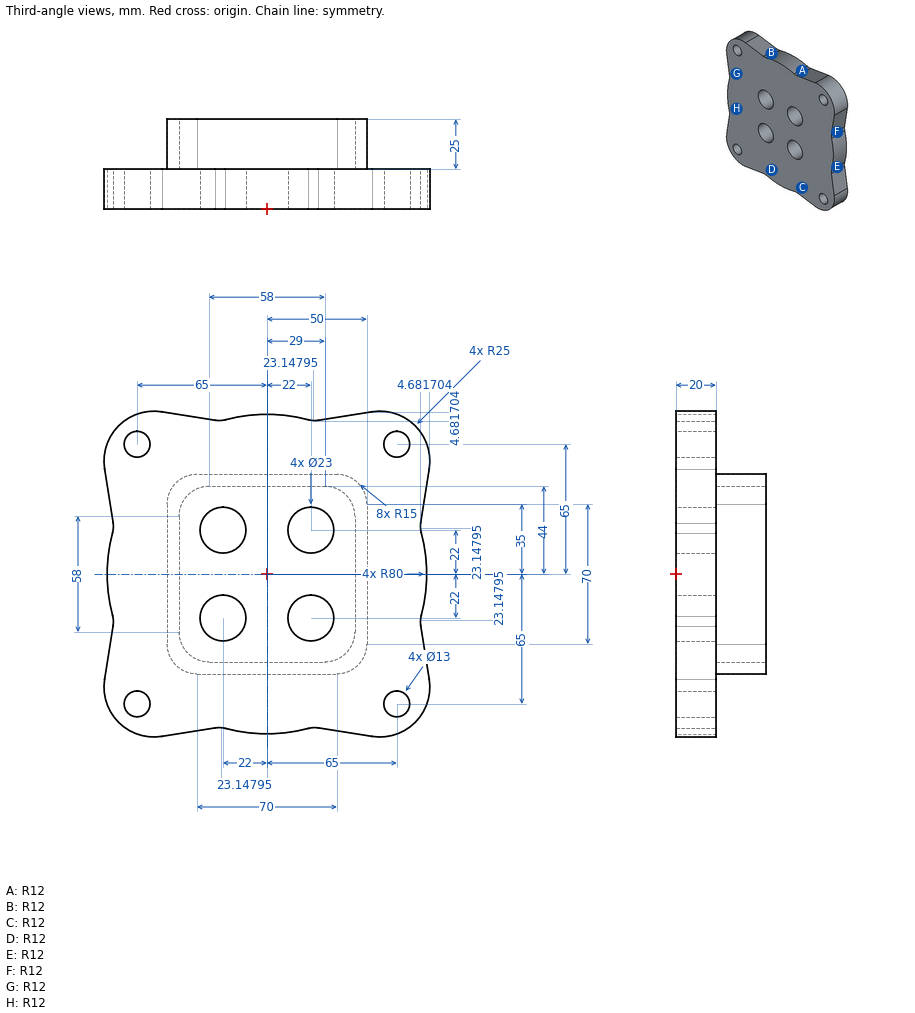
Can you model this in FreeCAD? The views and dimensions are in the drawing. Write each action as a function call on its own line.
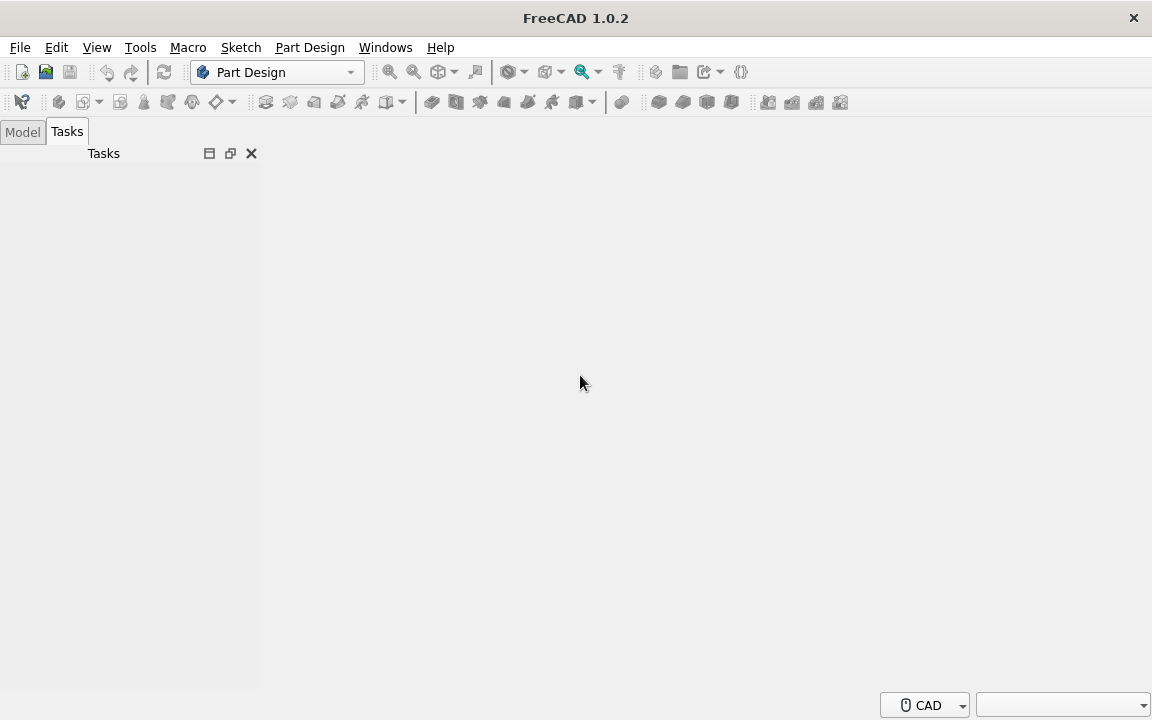
click(22, 72)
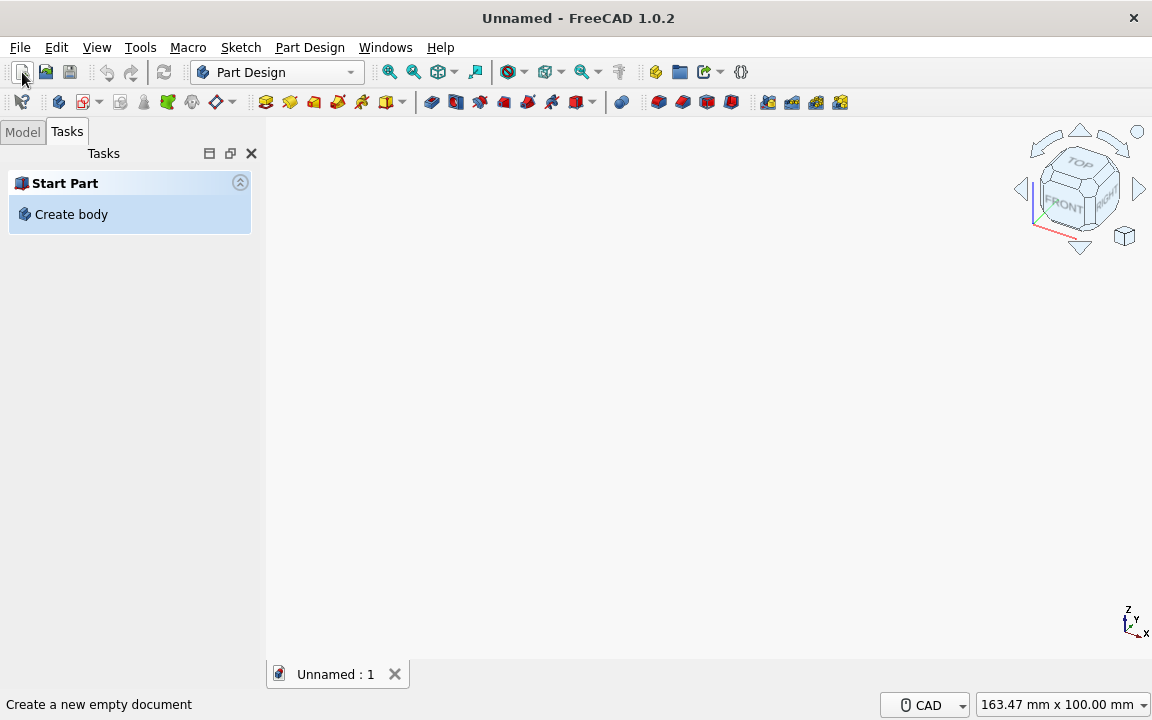
click(84, 102)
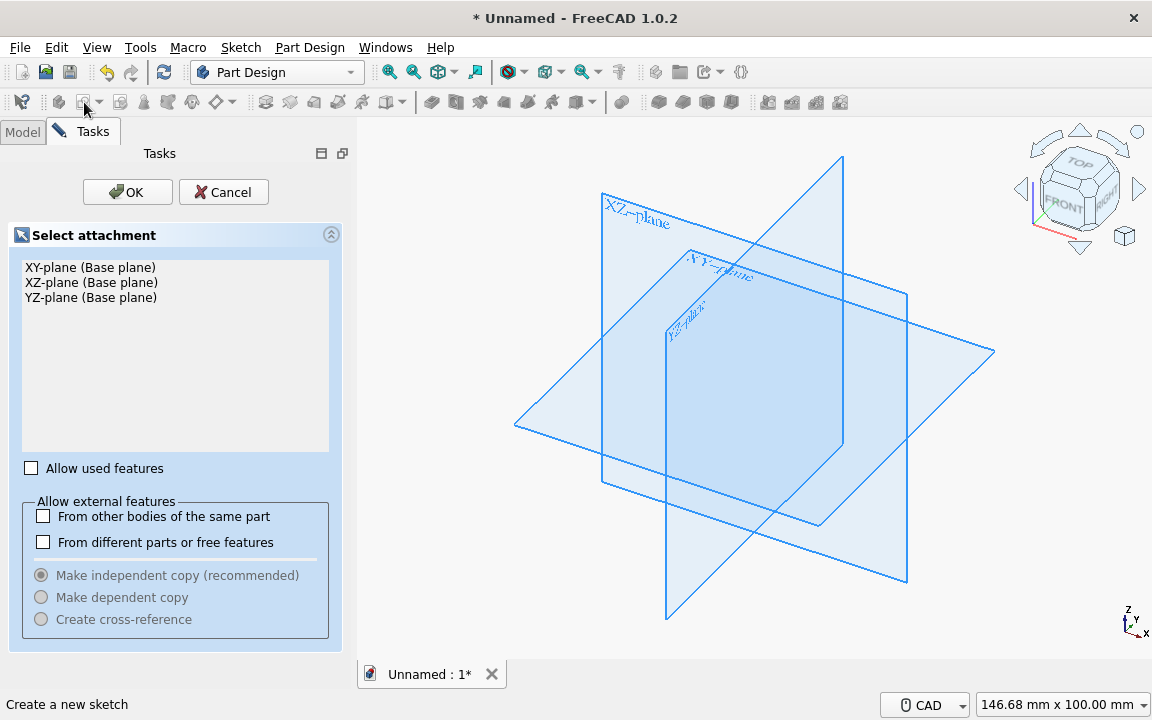
click(82, 282)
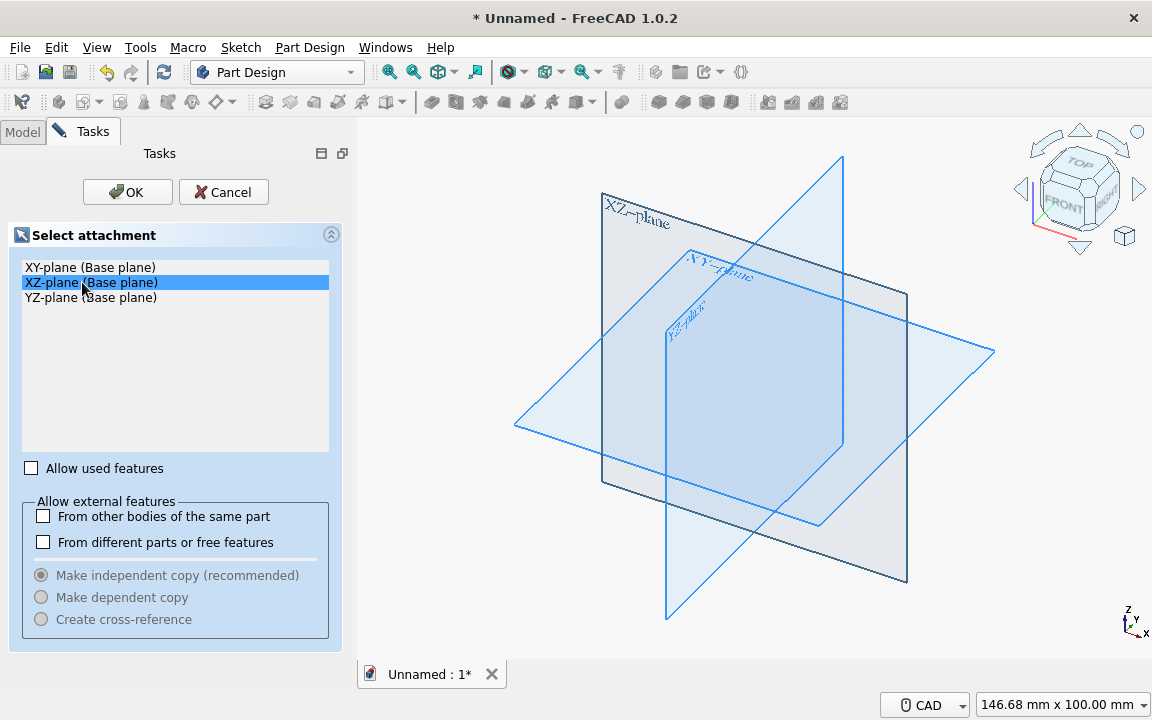
click(128, 192)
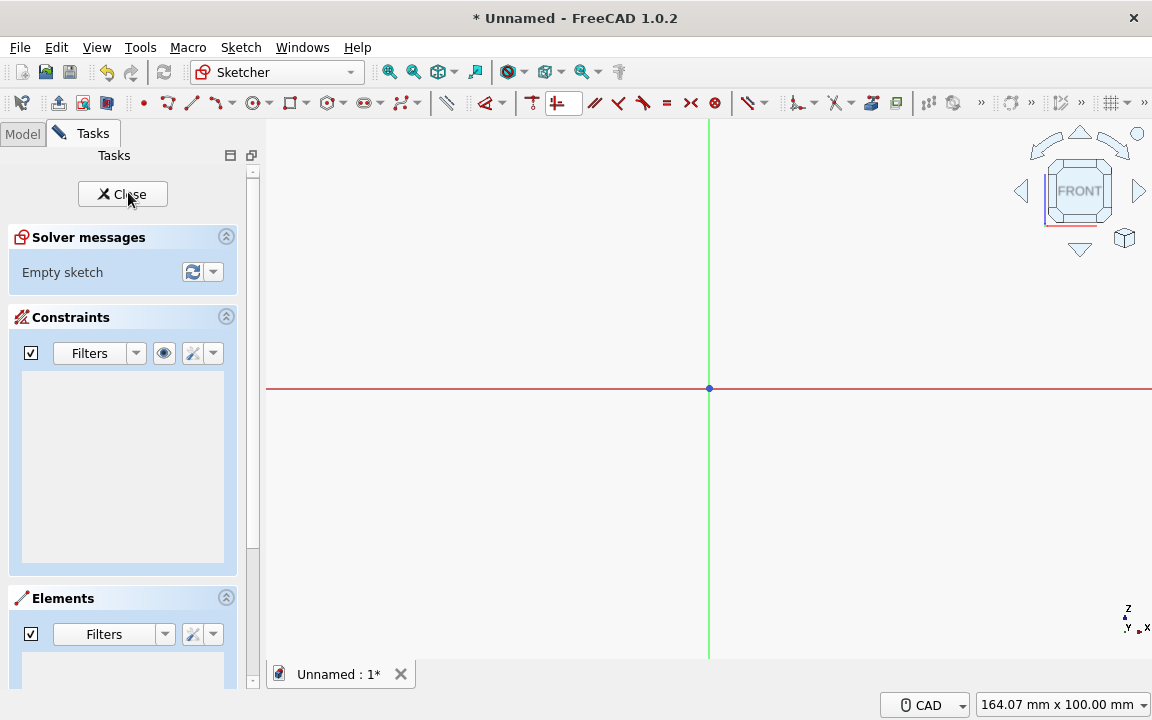
scroll(601, 389, down, 5)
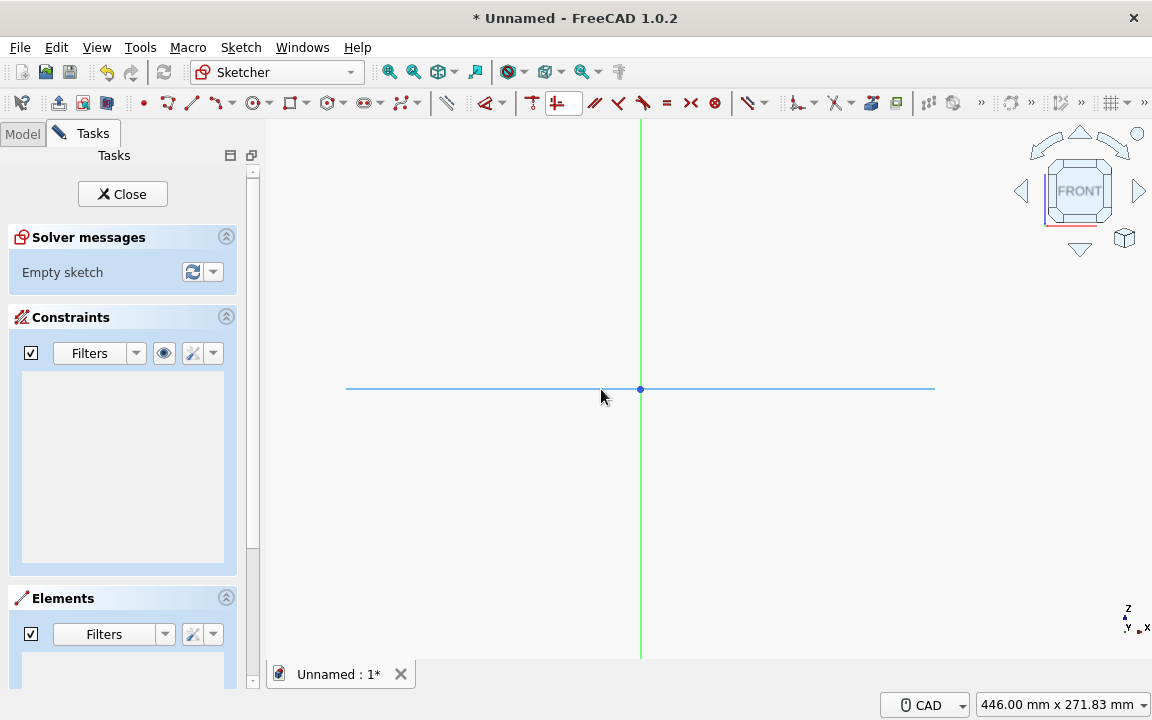
click(192, 104)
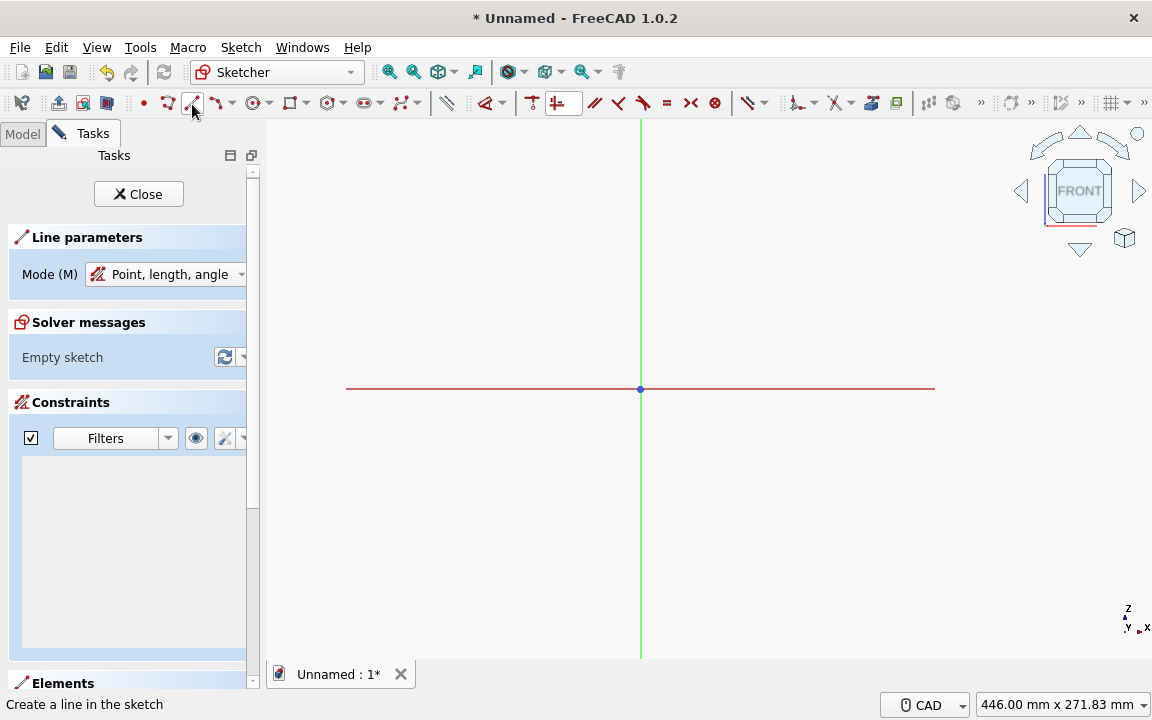
click(687, 237)
click(746, 228)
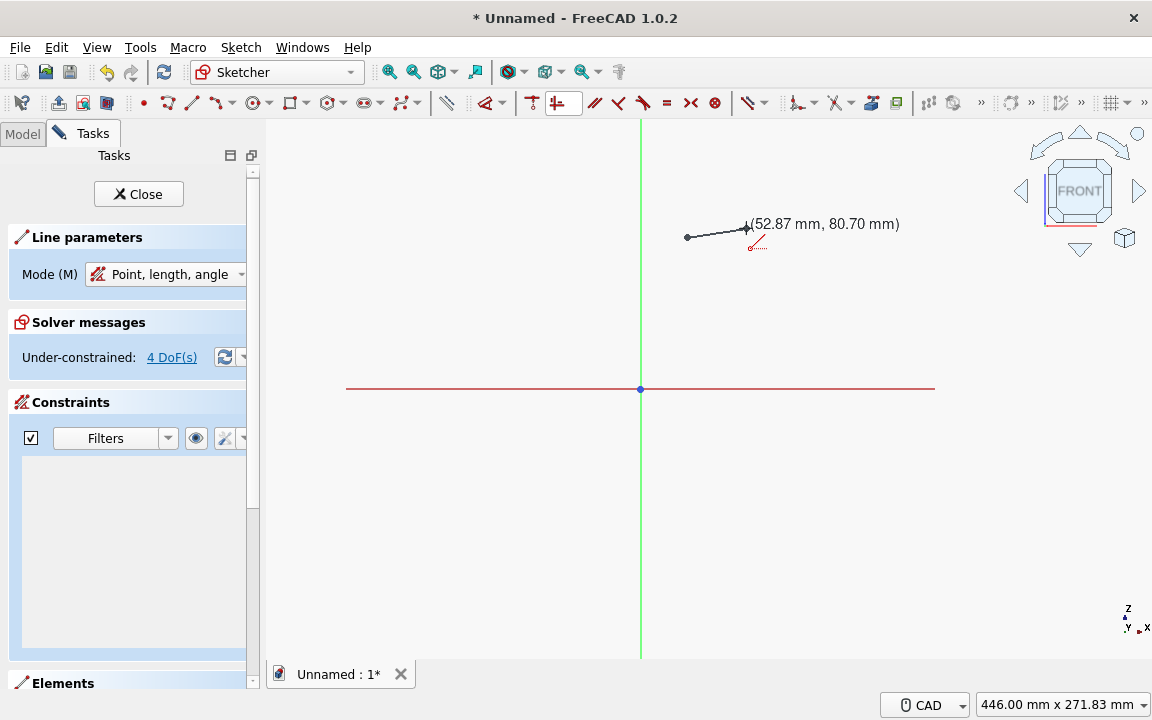
click(802, 285)
click(793, 343)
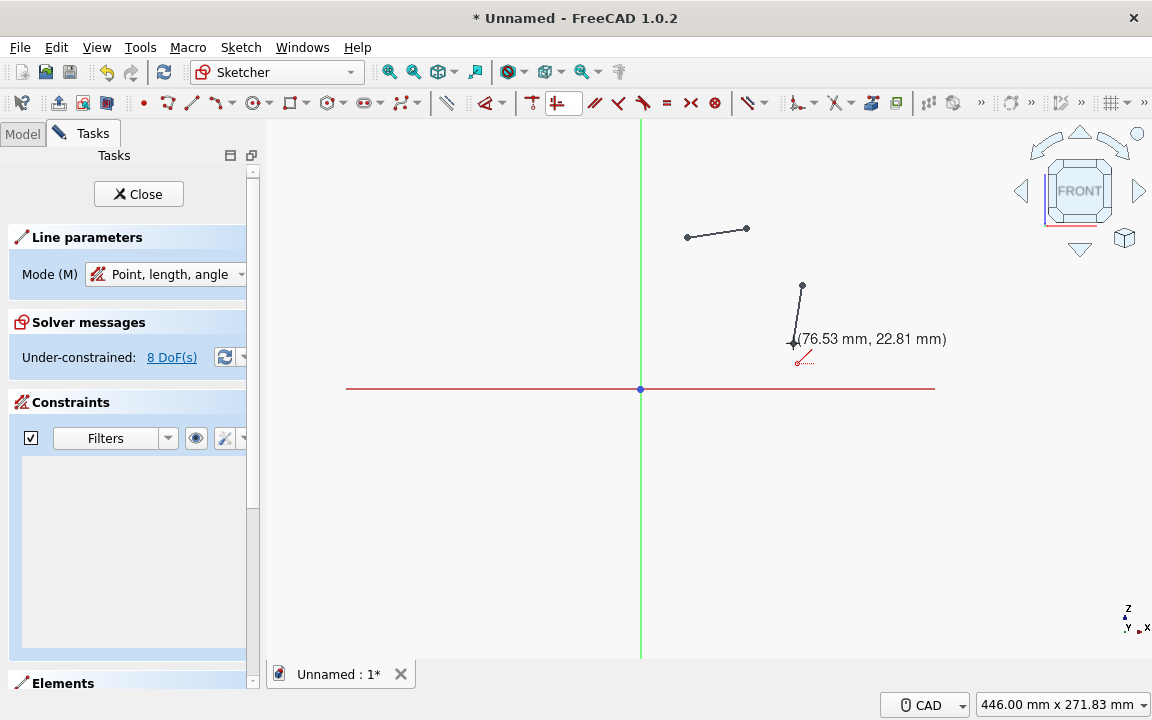
click(793, 435)
click(802, 494)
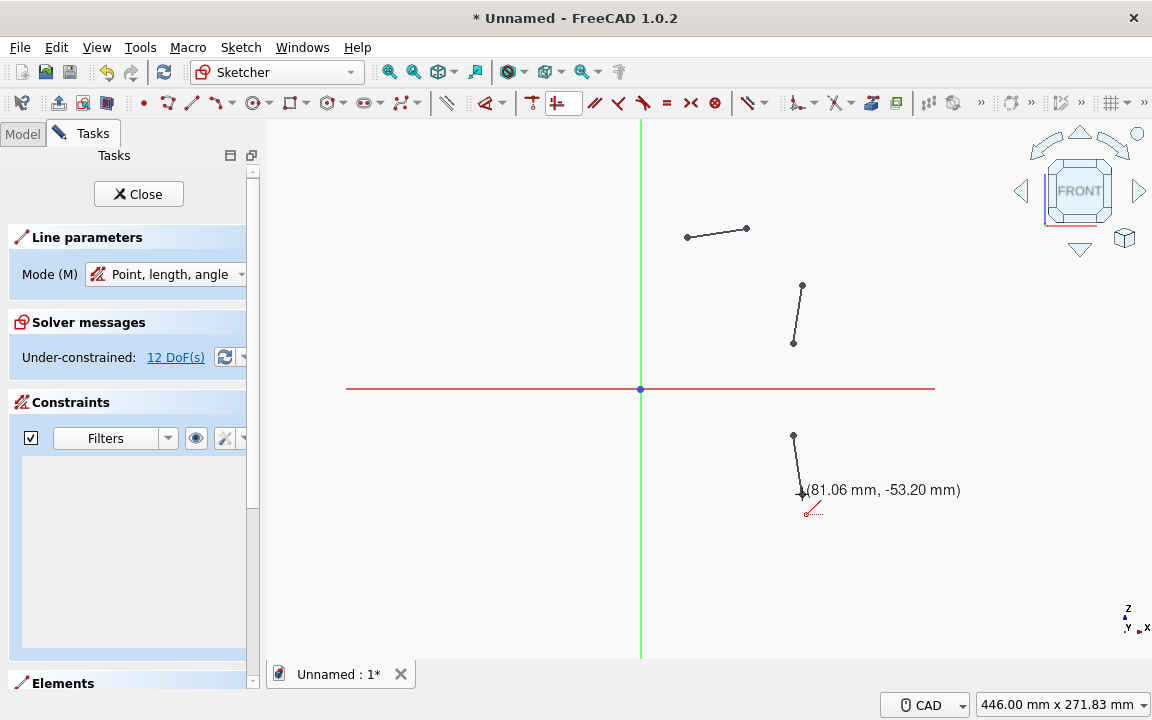
click(746, 551)
click(687, 541)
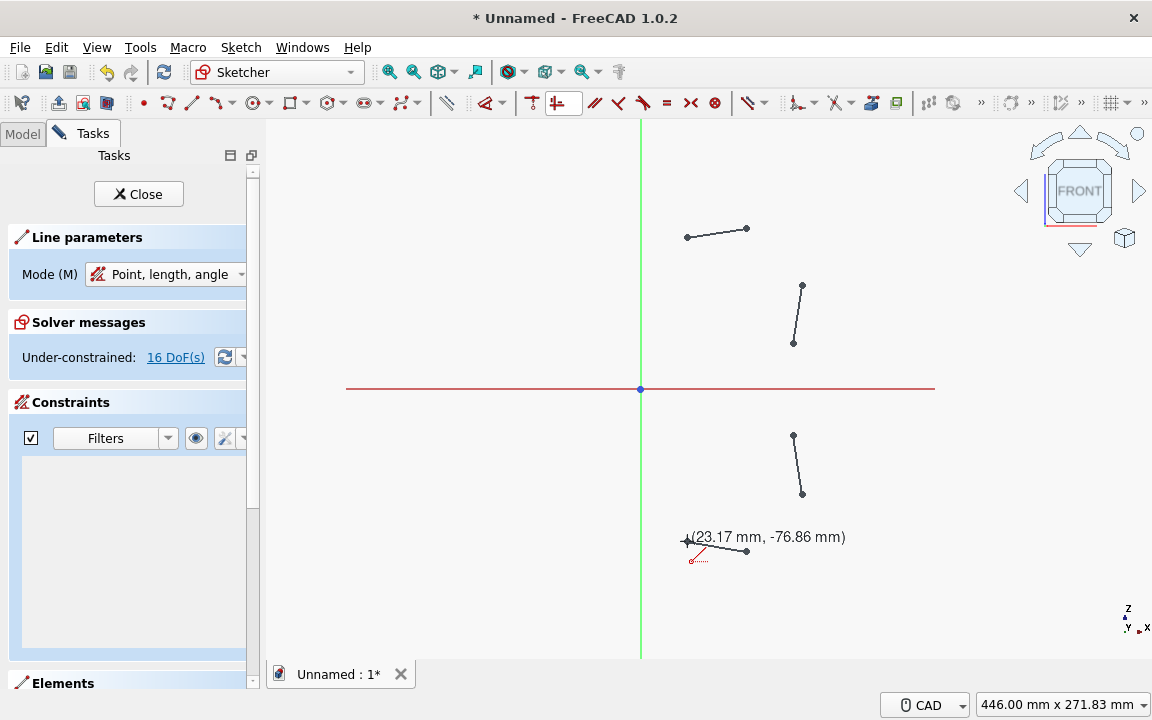
click(595, 541)
click(536, 551)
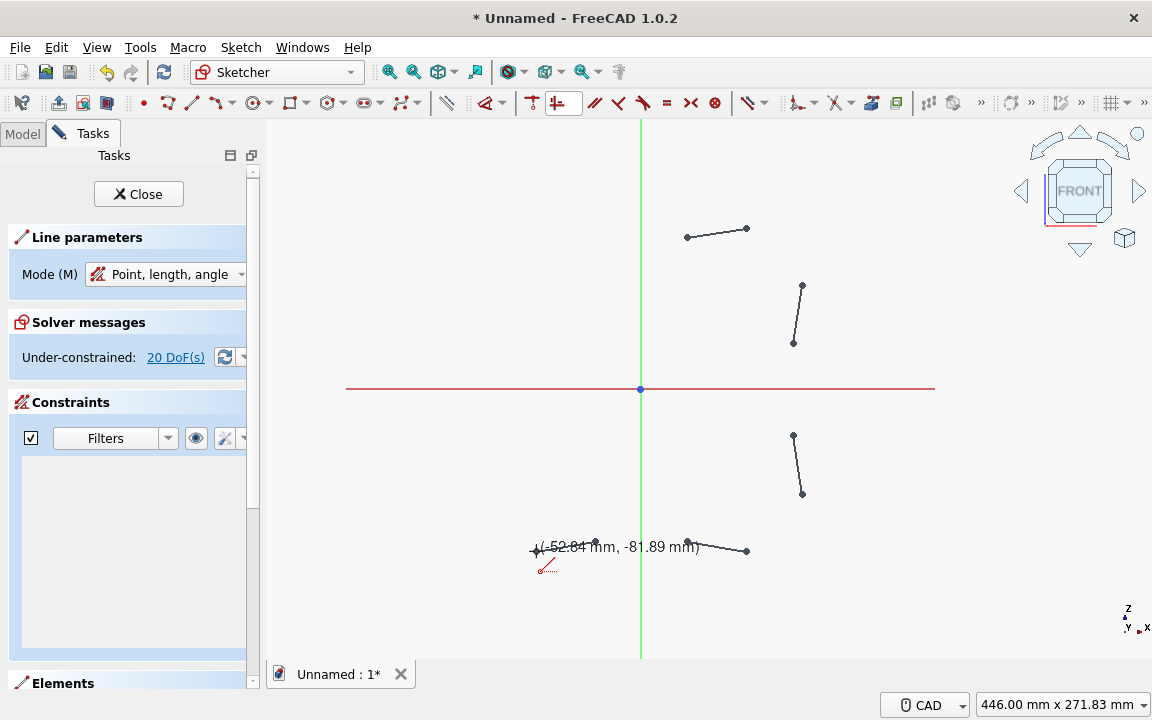
click(480, 494)
click(489, 435)